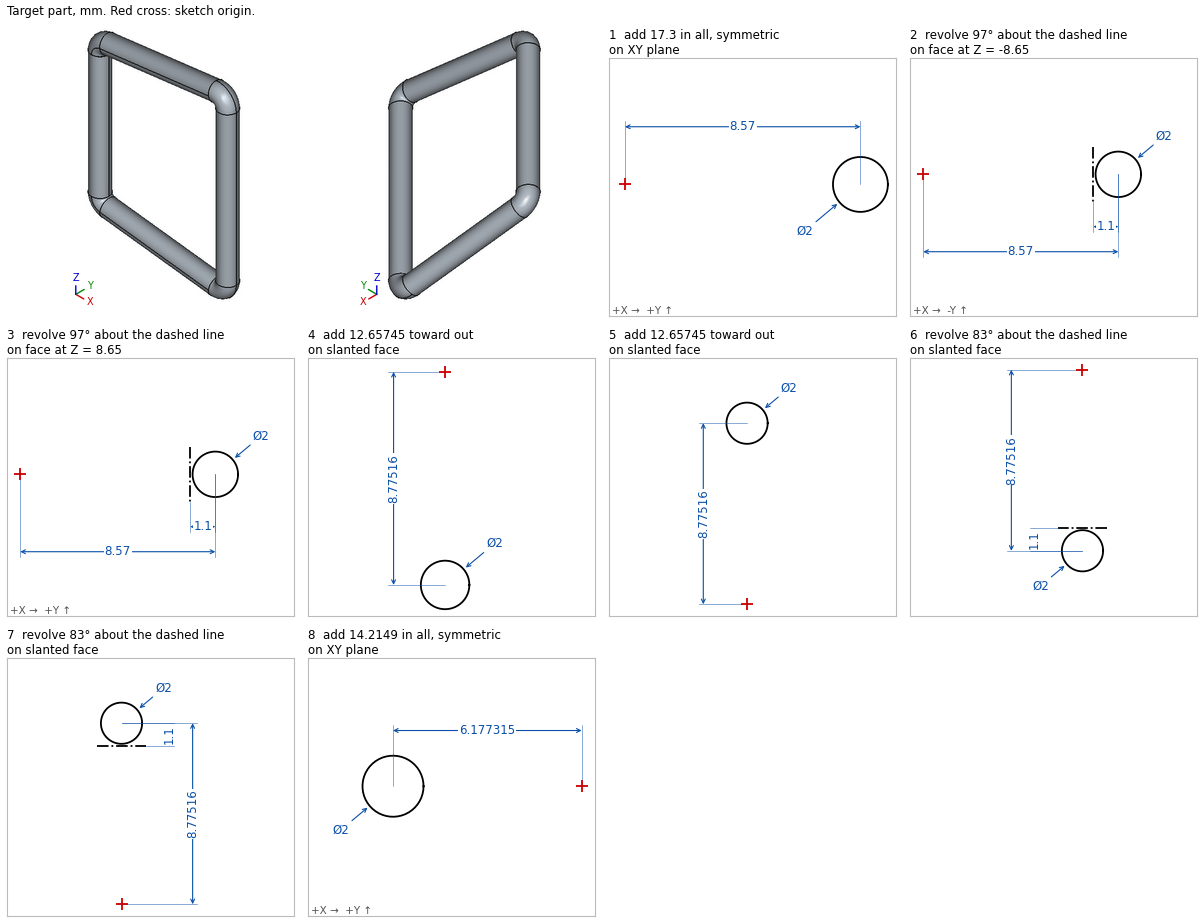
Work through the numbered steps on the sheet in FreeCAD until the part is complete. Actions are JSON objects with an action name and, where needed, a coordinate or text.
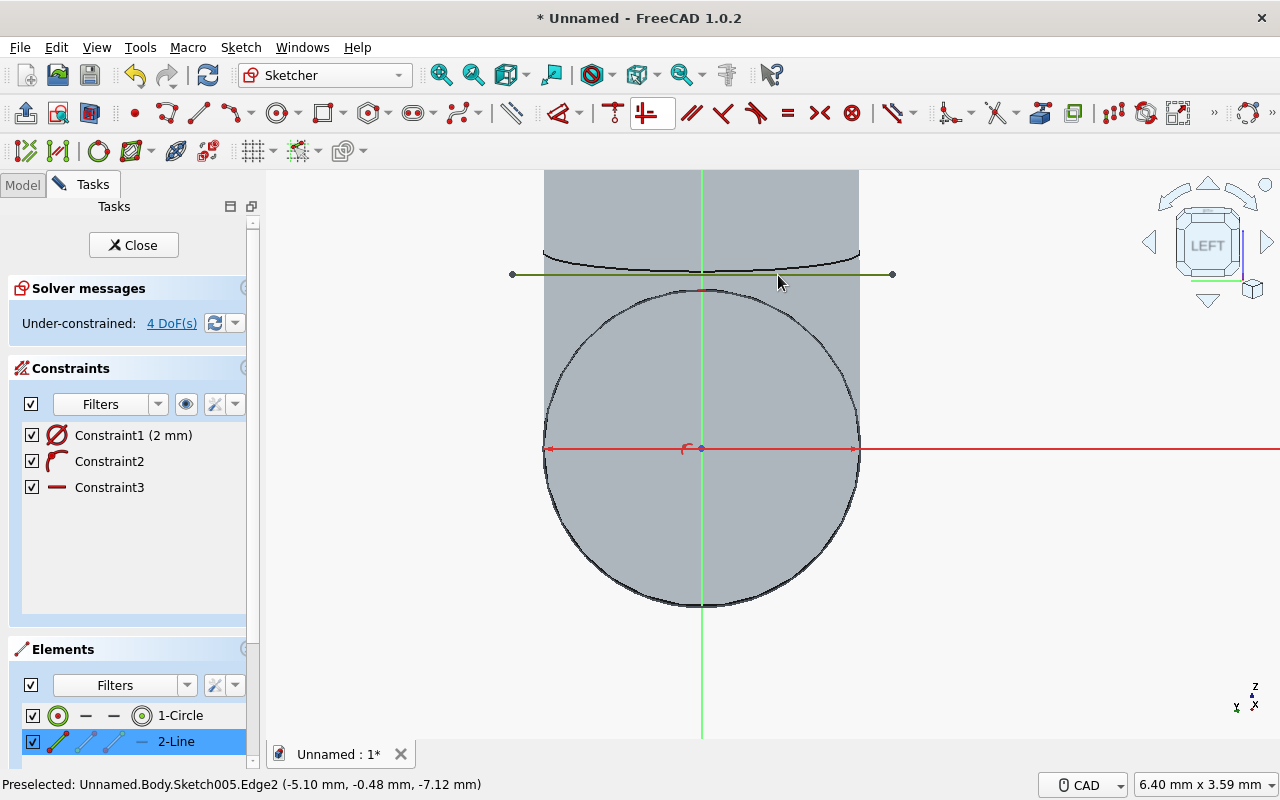
{"action": "left_click", "coordinate": [512, 114]}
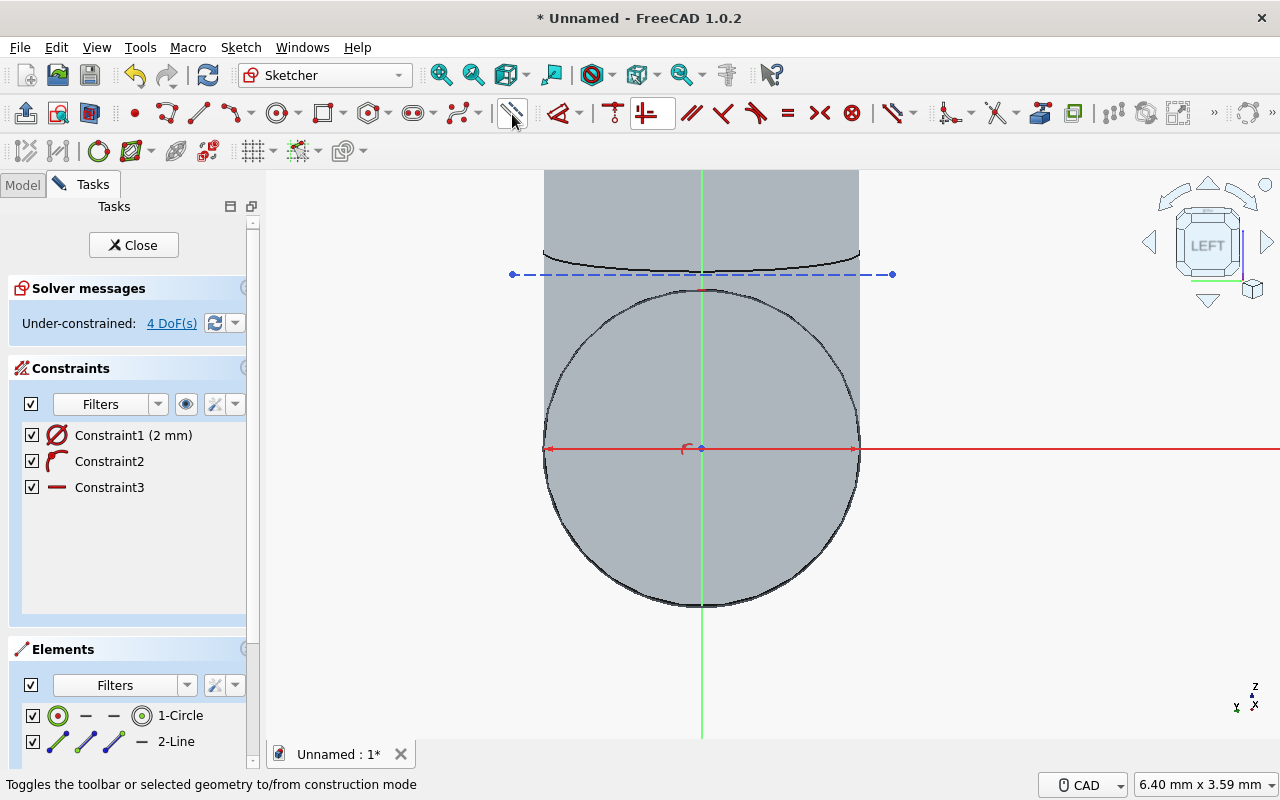
{"action": "left_click", "coordinate": [558, 114]}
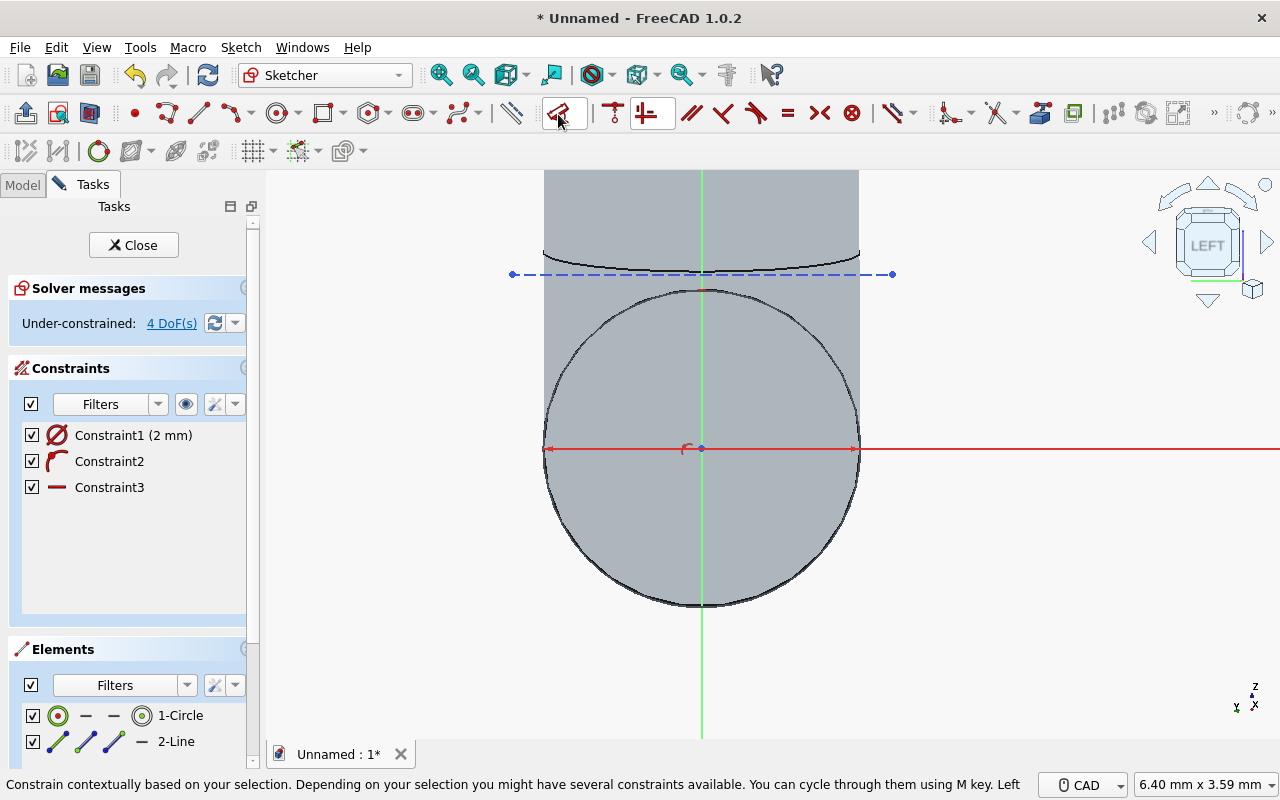
{"action": "left_click", "coordinate": [512, 275]}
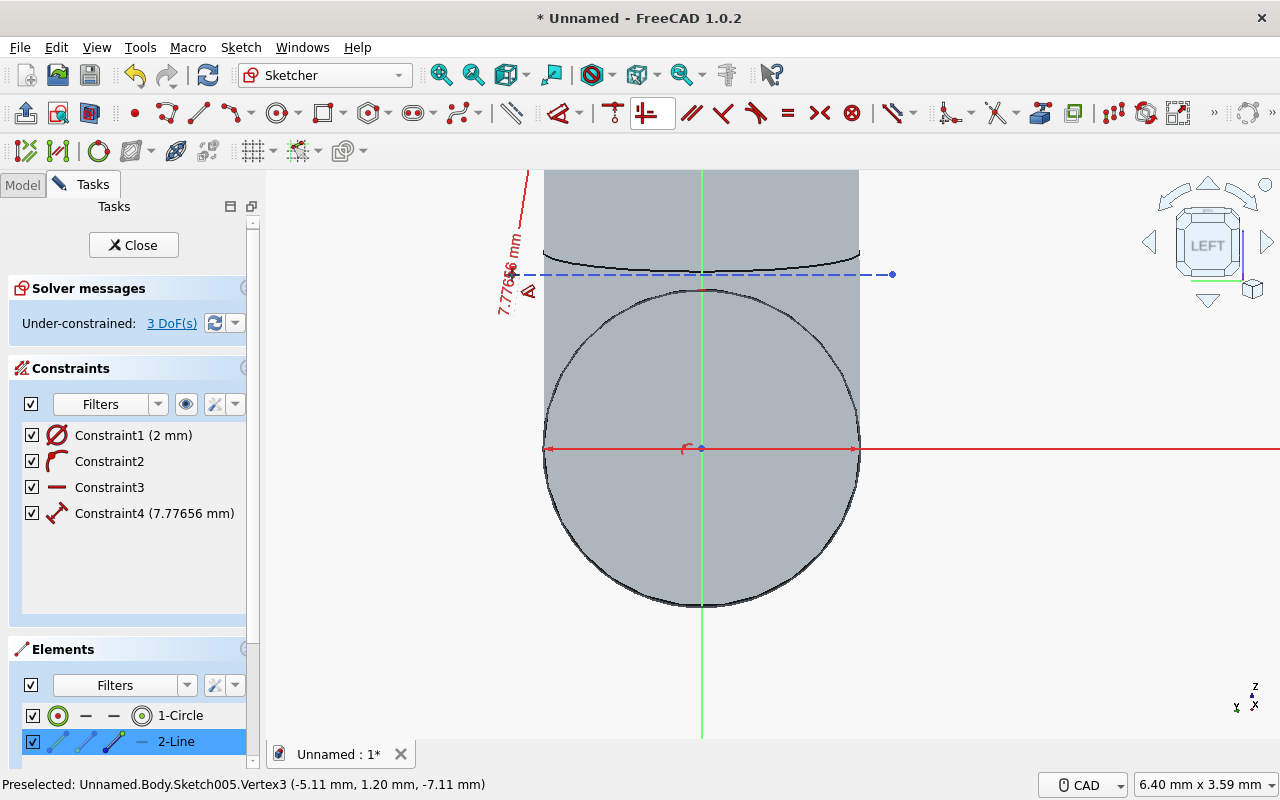
{"action": "left_click", "coordinate": [702, 449]}
{"action": "left_click", "coordinate": [478, 362]}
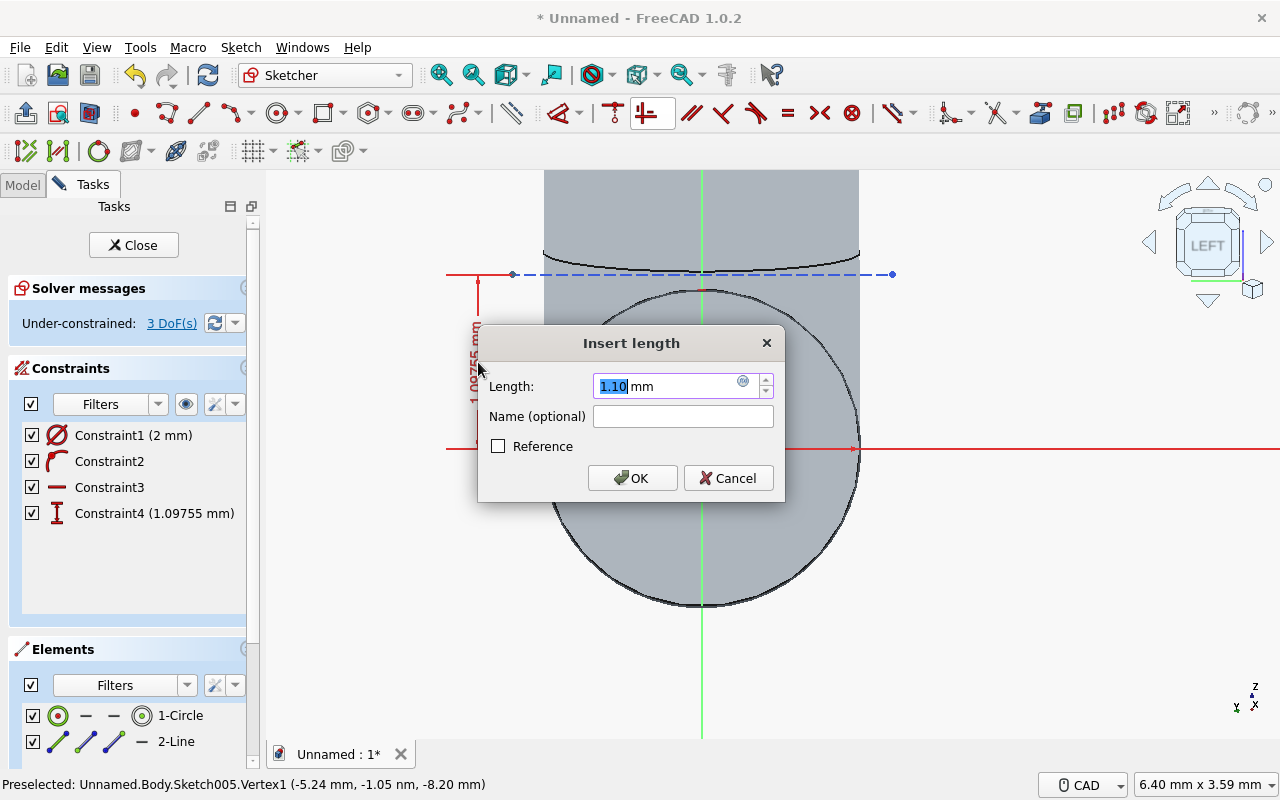
{"action": "type", "text": "1.1"}
{"action": "key", "text": "Return"}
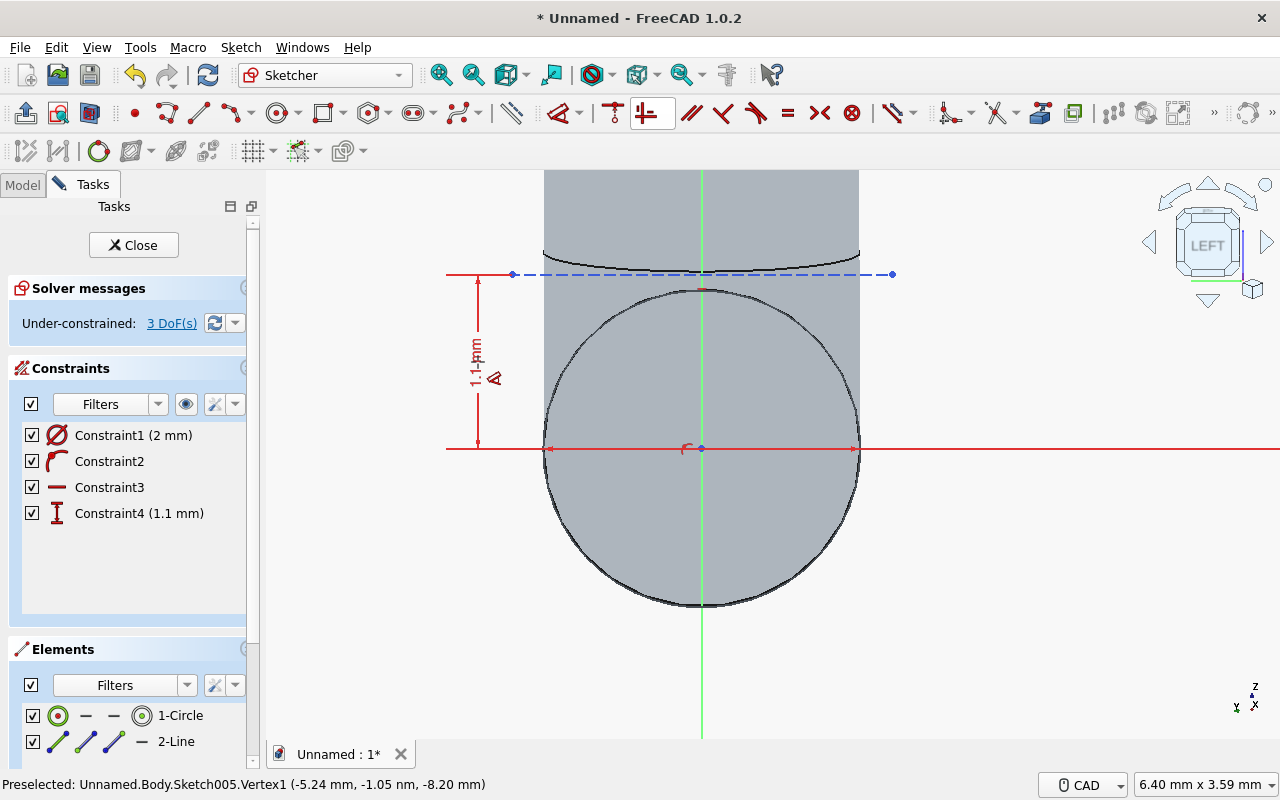
{"action": "left_click", "coordinate": [702, 449]}
{"action": "left_click", "coordinate": [668, 323]}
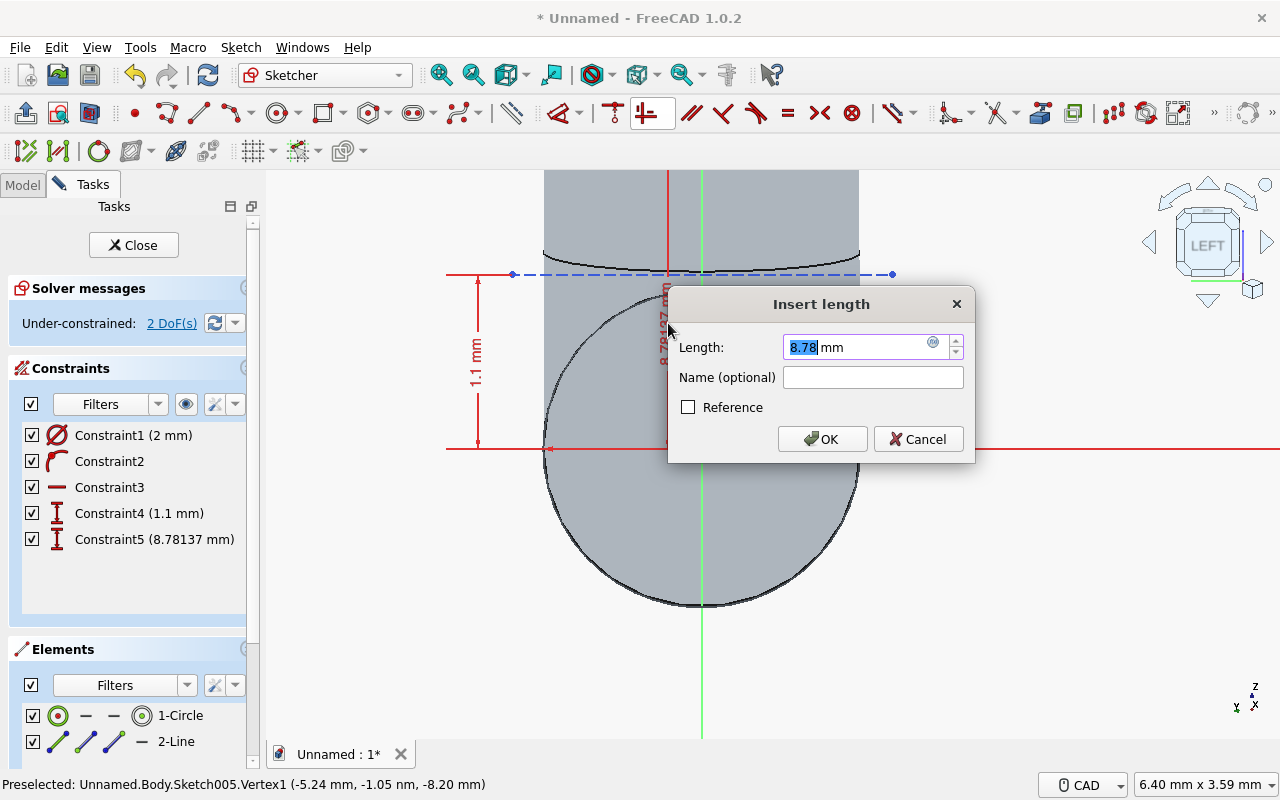
{"action": "type", "text": "8.77516"}
{"action": "key", "text": "Return"}
{"action": "key", "text": "Escape"}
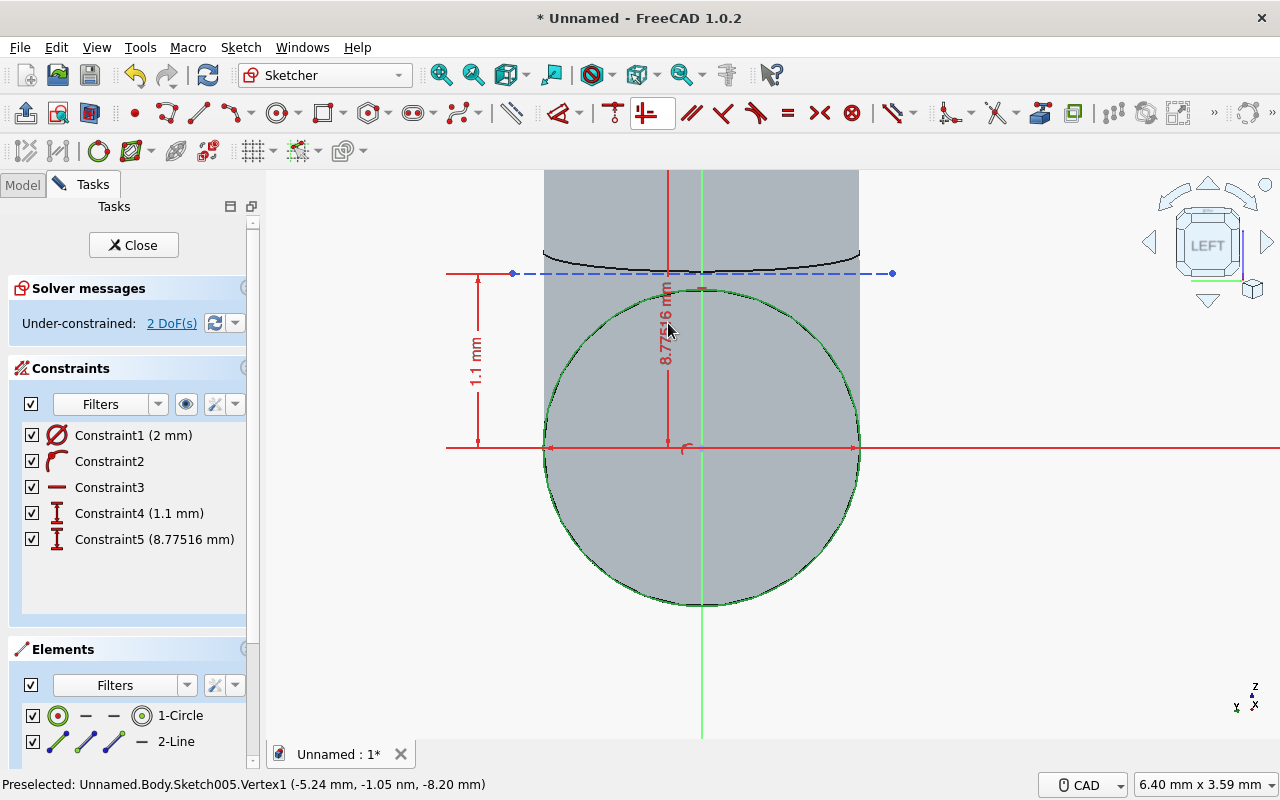
{"action": "left_click", "coordinate": [134, 245]}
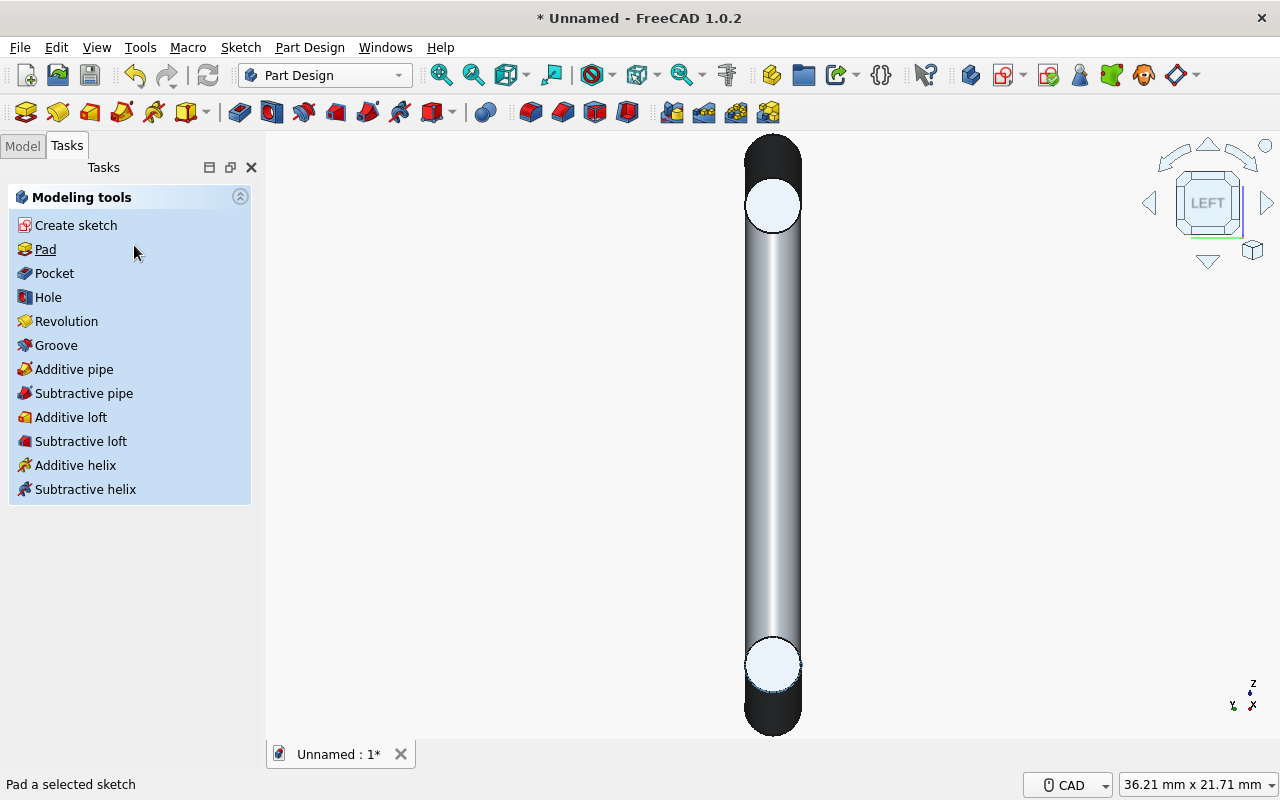
{"action": "left_click", "coordinate": [58, 112]}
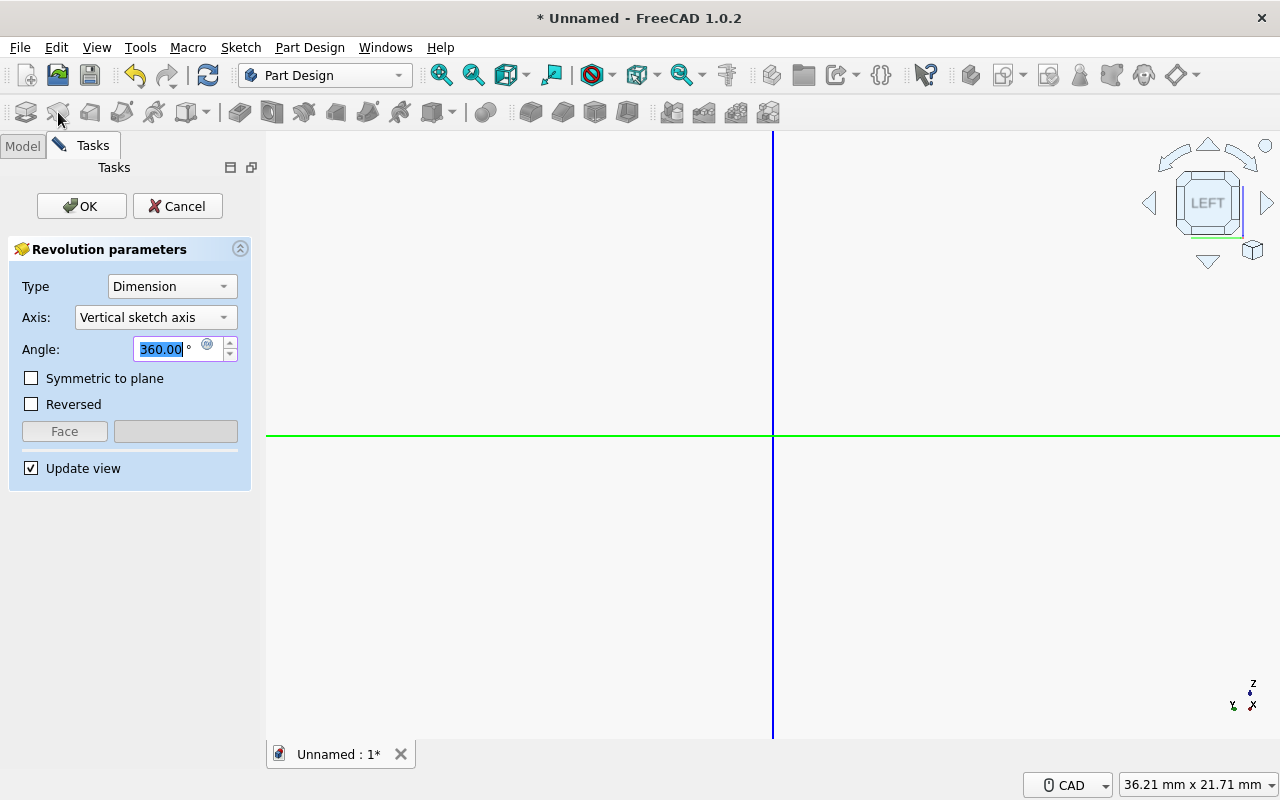
{"action": "left_click", "coordinate": [156, 318]}